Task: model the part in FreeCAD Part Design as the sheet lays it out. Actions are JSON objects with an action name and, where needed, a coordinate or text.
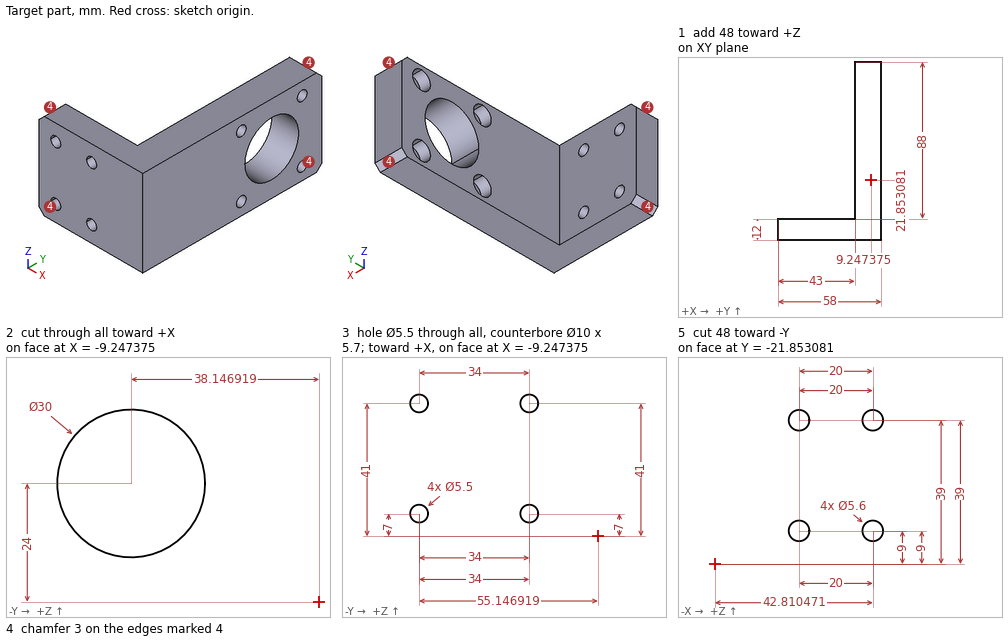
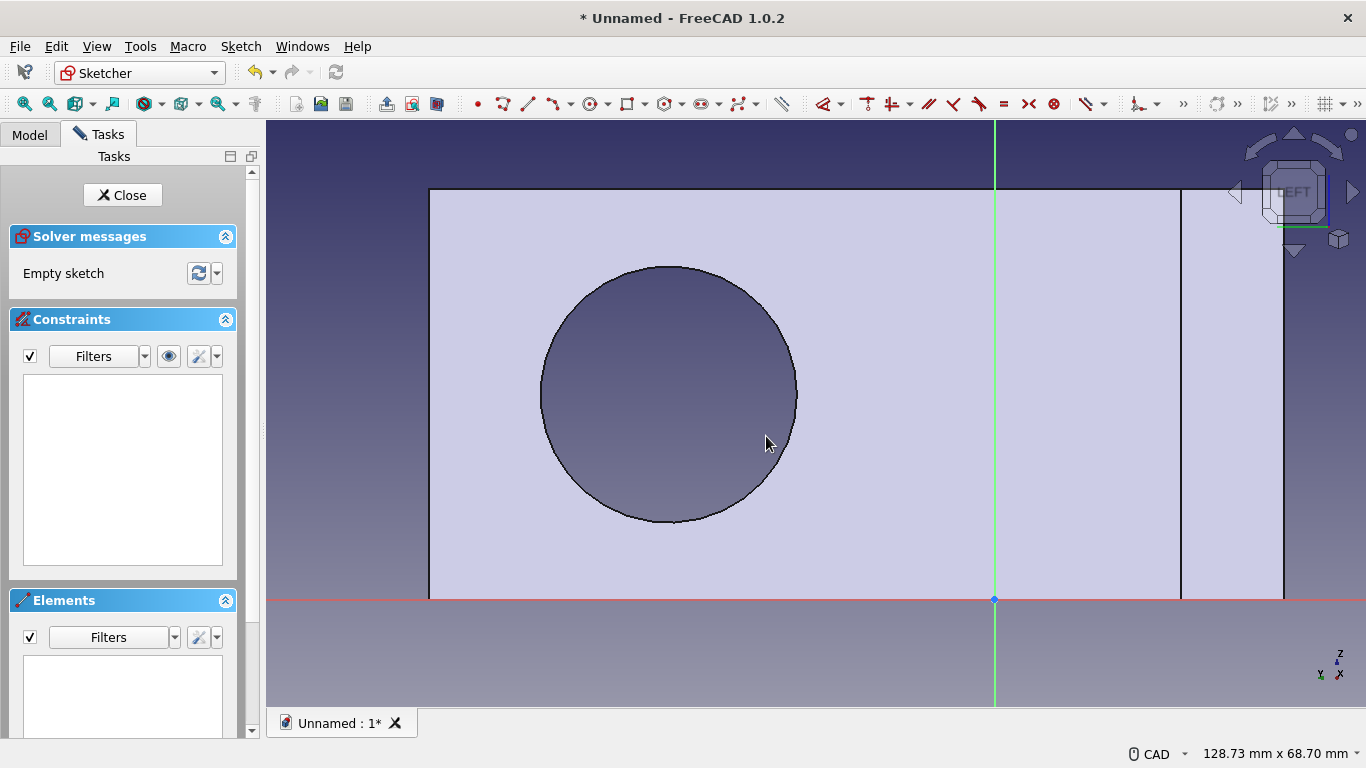
{"action": "left_click", "coordinate": [590, 104]}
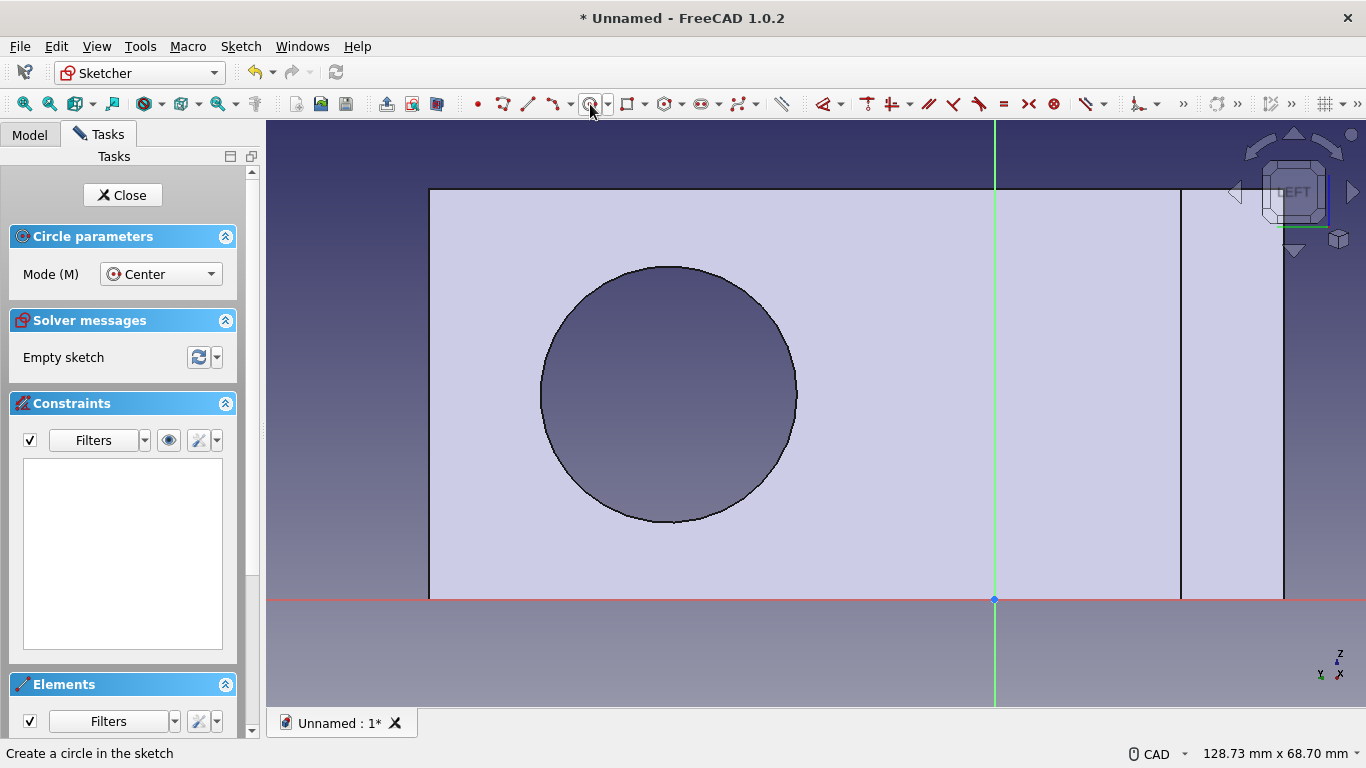
{"action": "left_click", "coordinate": [523, 540]}
{"action": "left_click", "coordinate": [540, 523]}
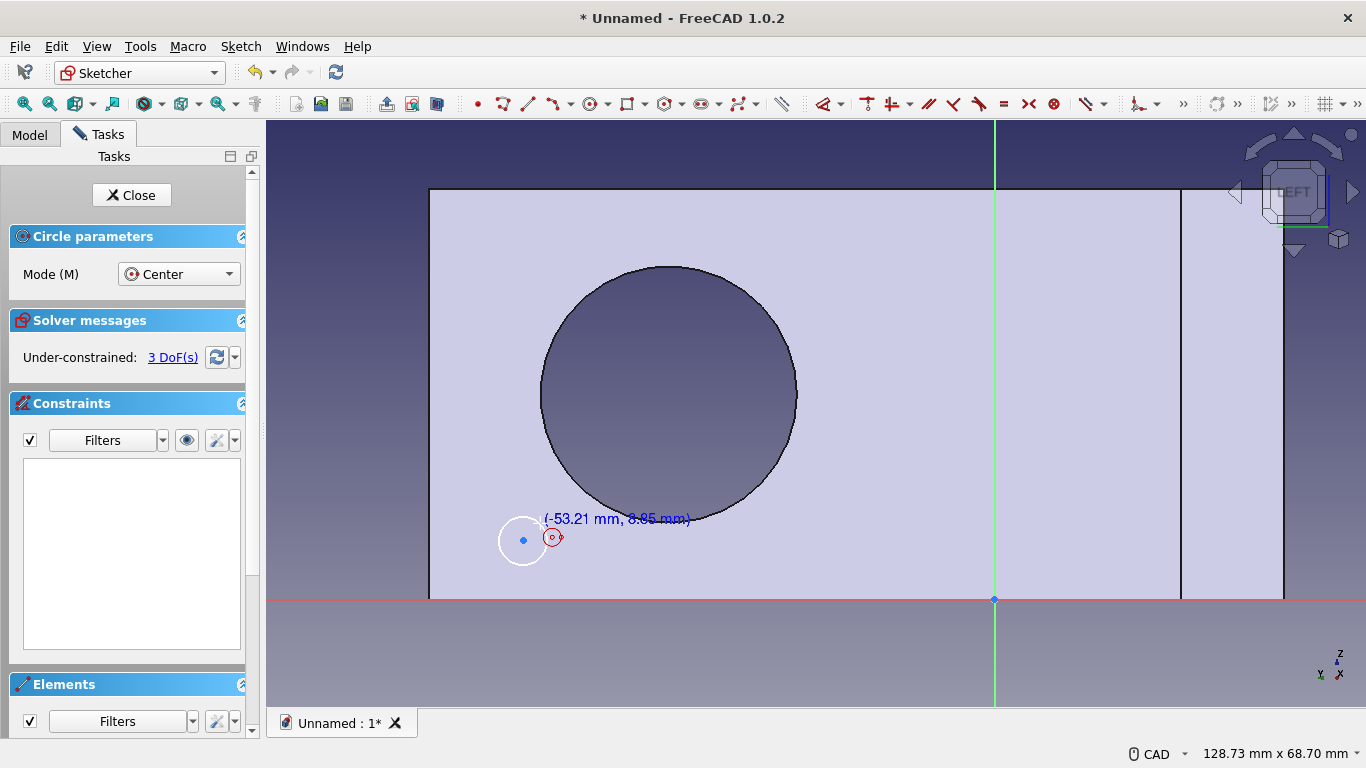
{"action": "left_click", "coordinate": [523, 249]}
{"action": "left_click", "coordinate": [540, 233]}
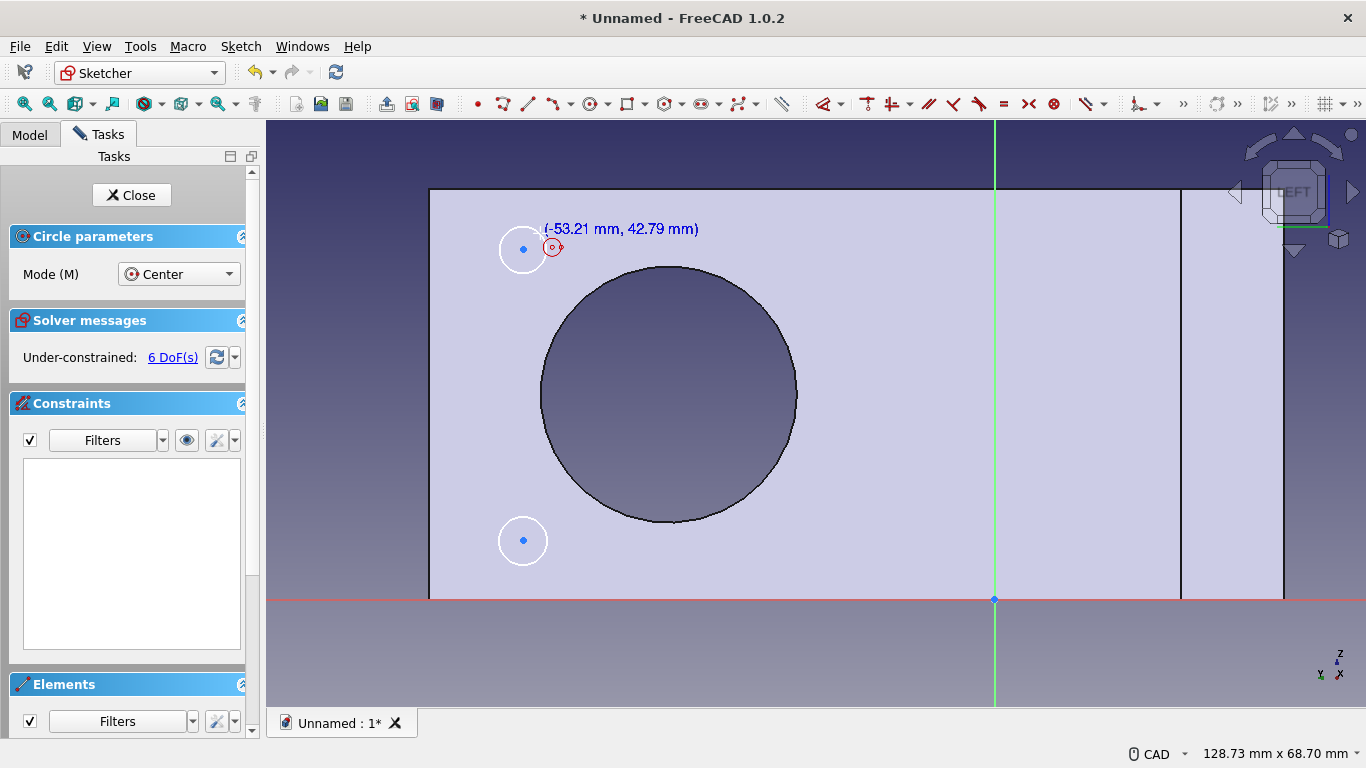
{"action": "left_click", "coordinate": [814, 249]}
{"action": "left_click", "coordinate": [831, 233]}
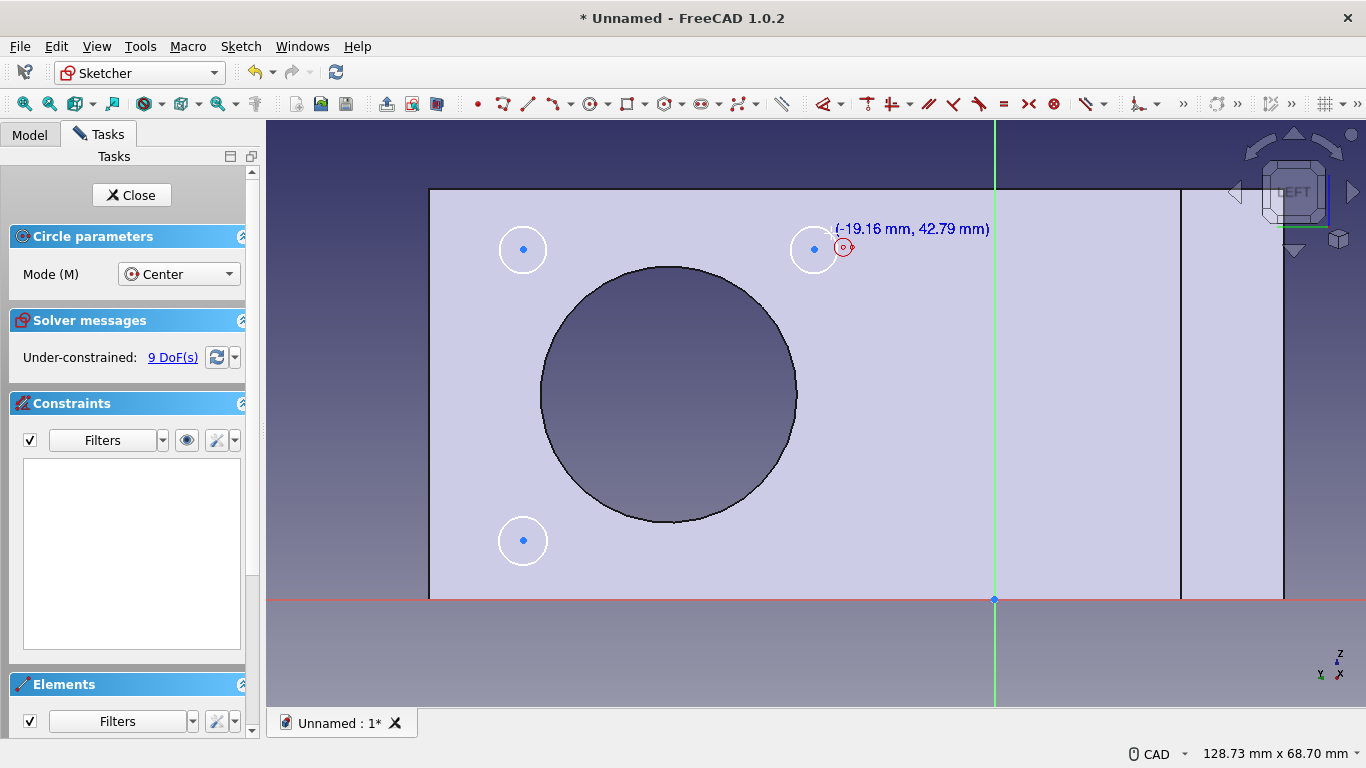
{"action": "left_click", "coordinate": [814, 540]}
{"action": "left_click", "coordinate": [831, 523]}
{"action": "key", "text": "Escape"}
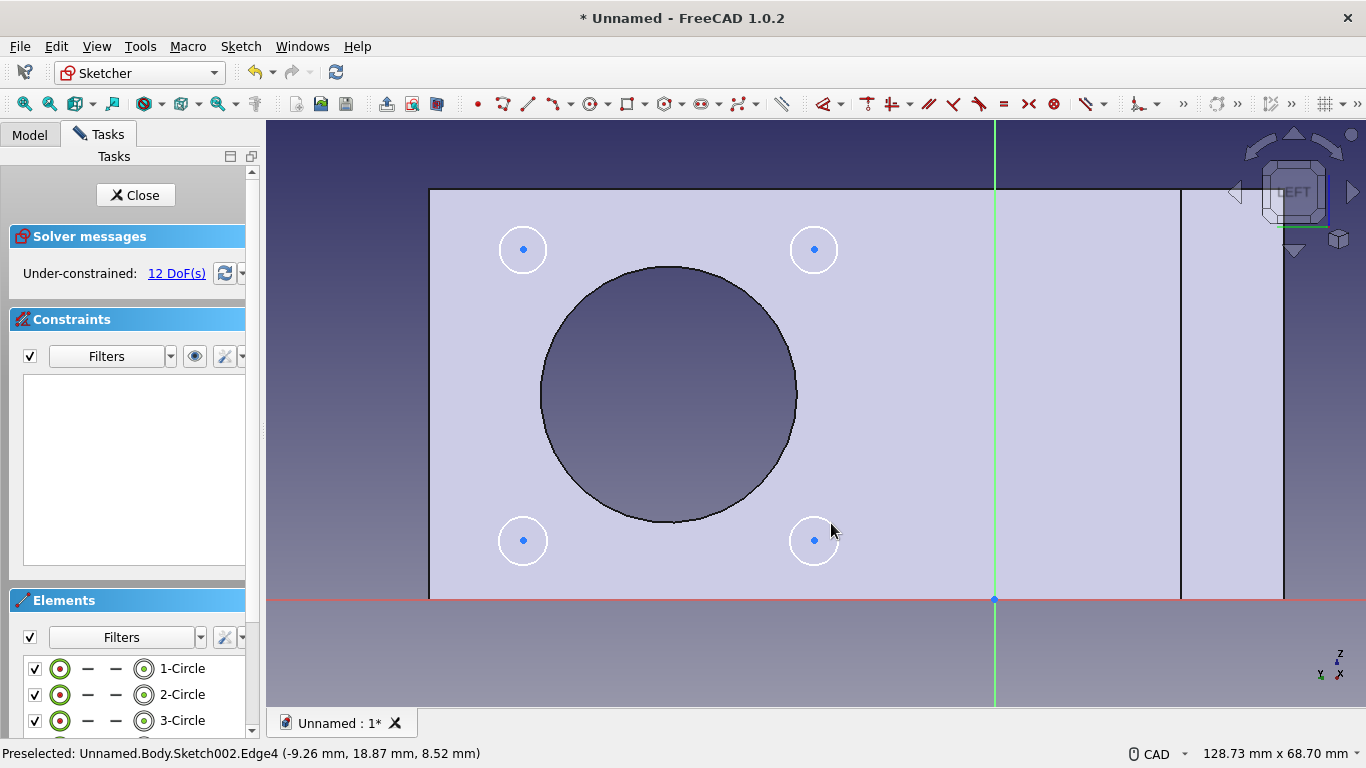
{"action": "left_click", "coordinate": [540, 524]}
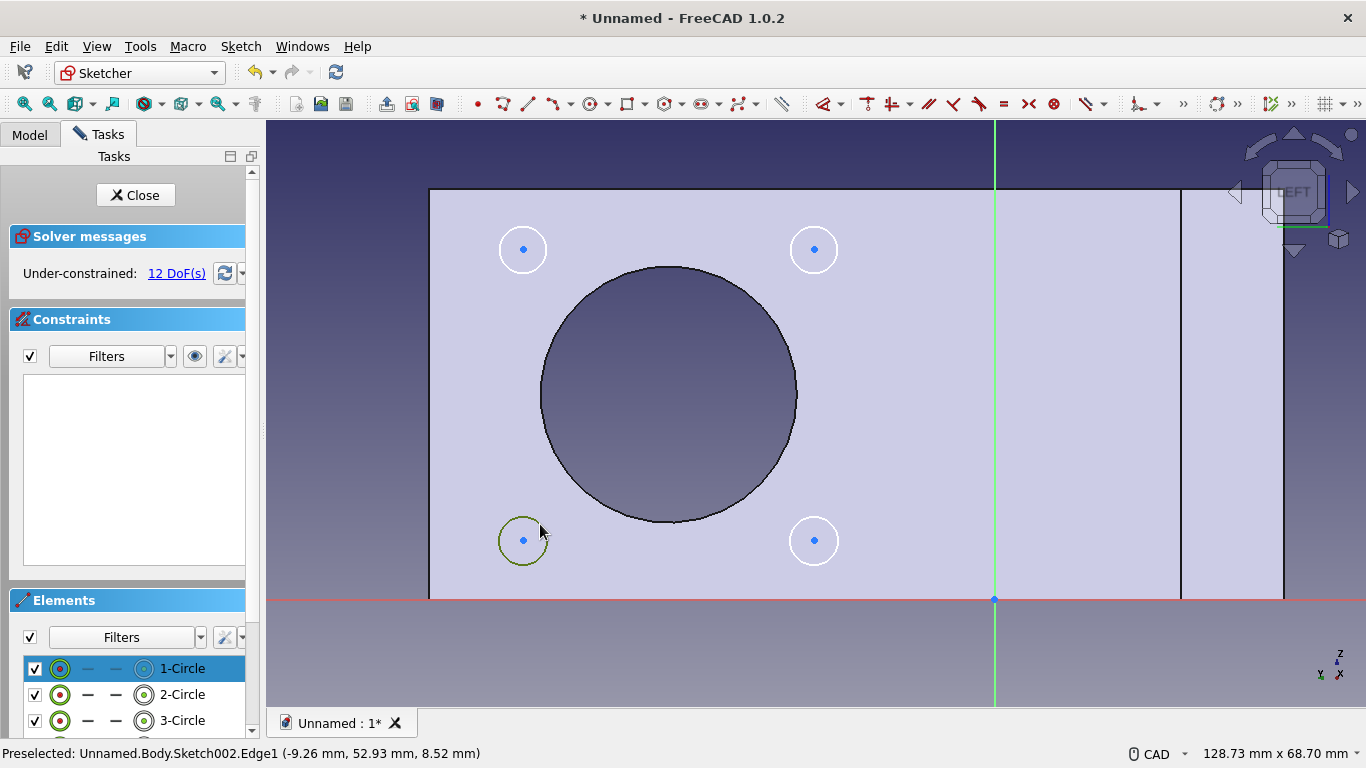
{"action": "left_click", "coordinate": [539, 233]}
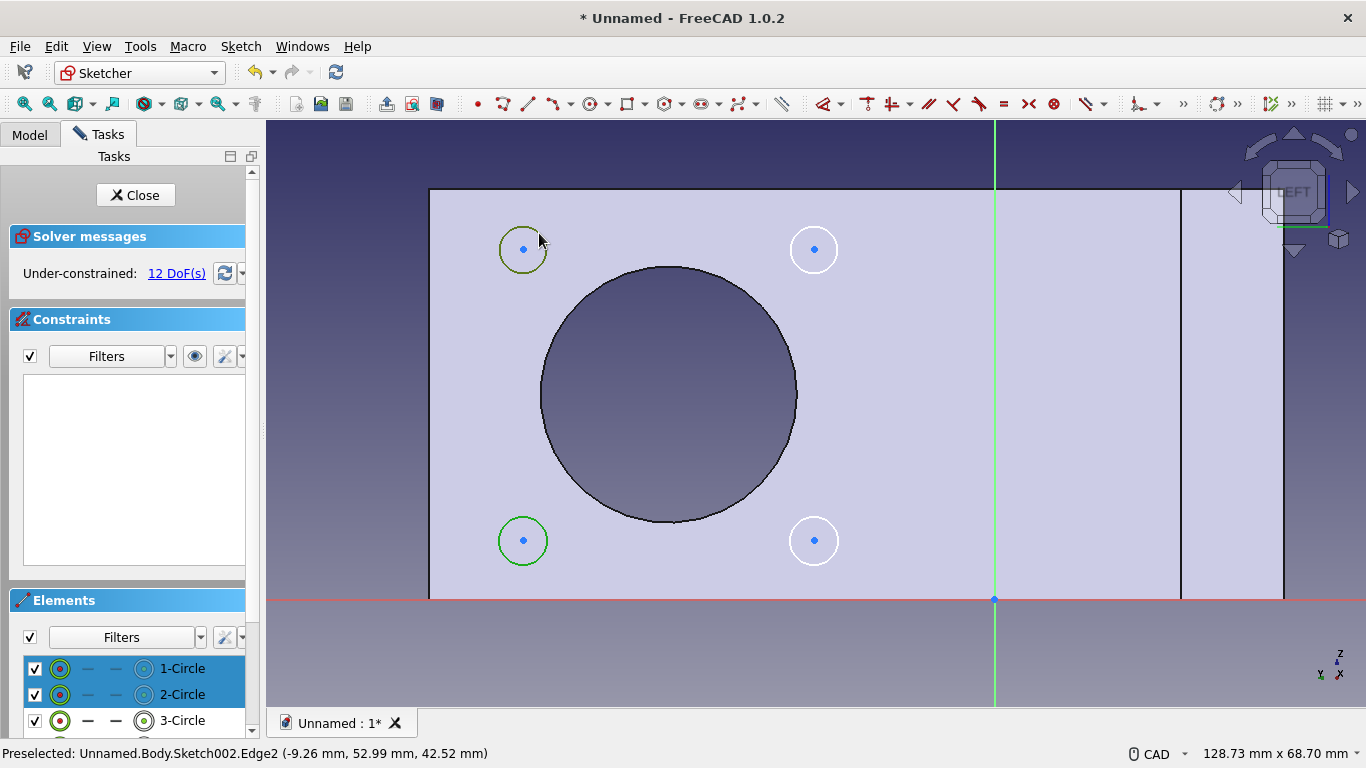
{"action": "left_click", "coordinate": [830, 233]}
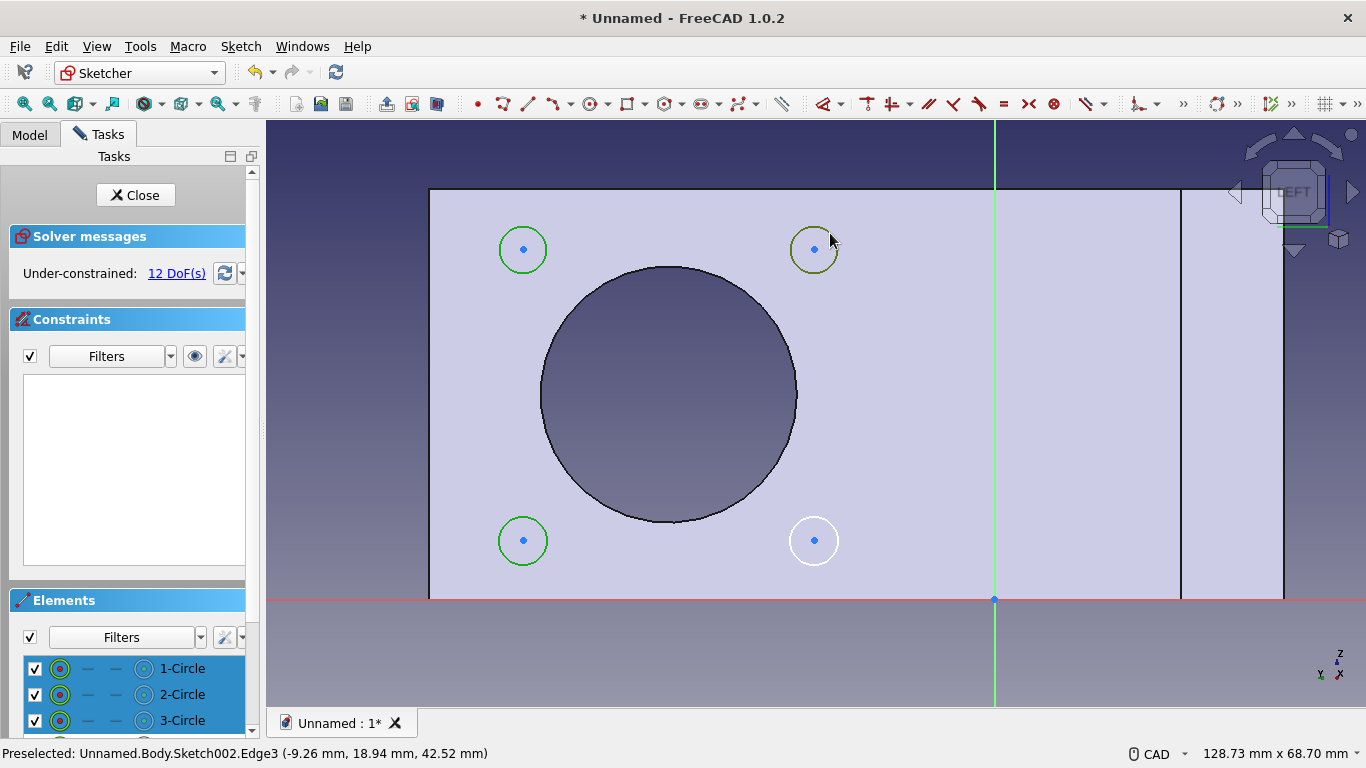
{"action": "left_click", "coordinate": [831, 524]}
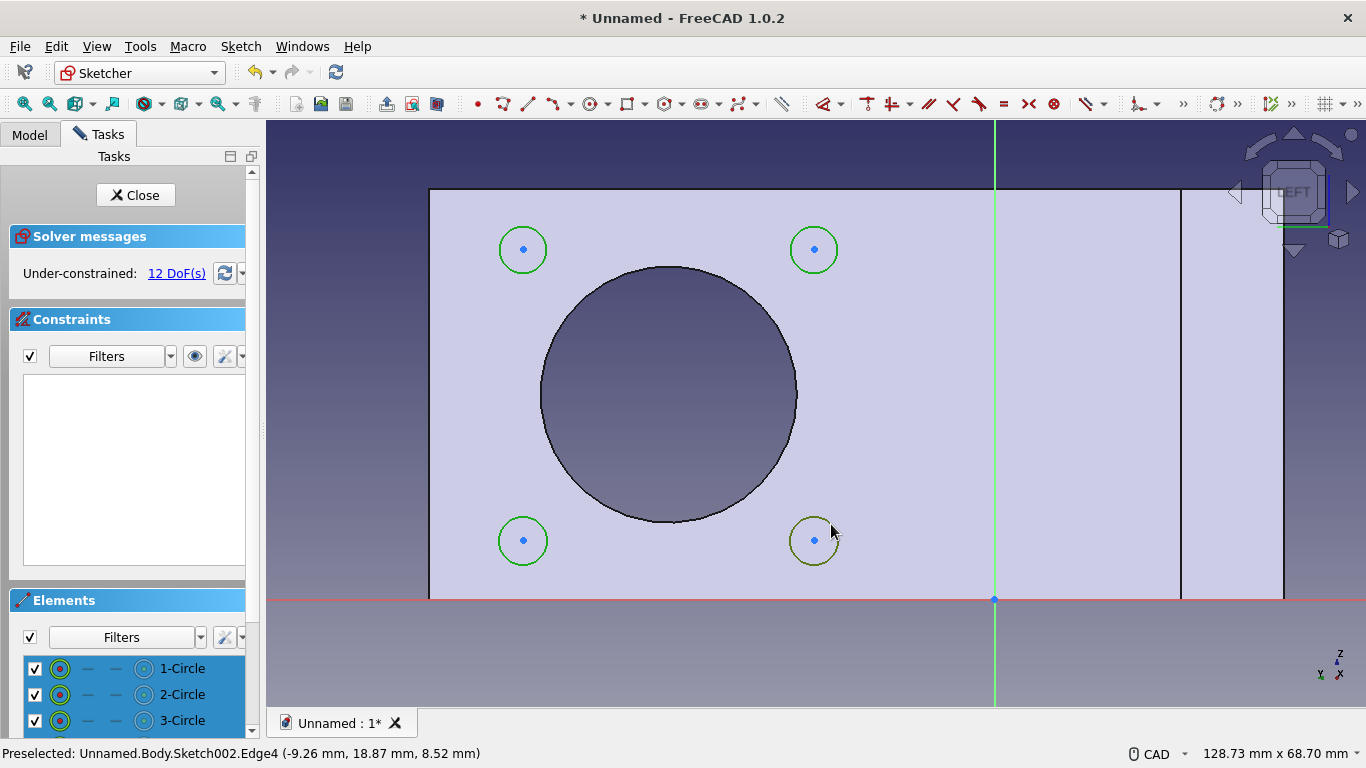
{"action": "left_click", "coordinate": [1004, 104]}